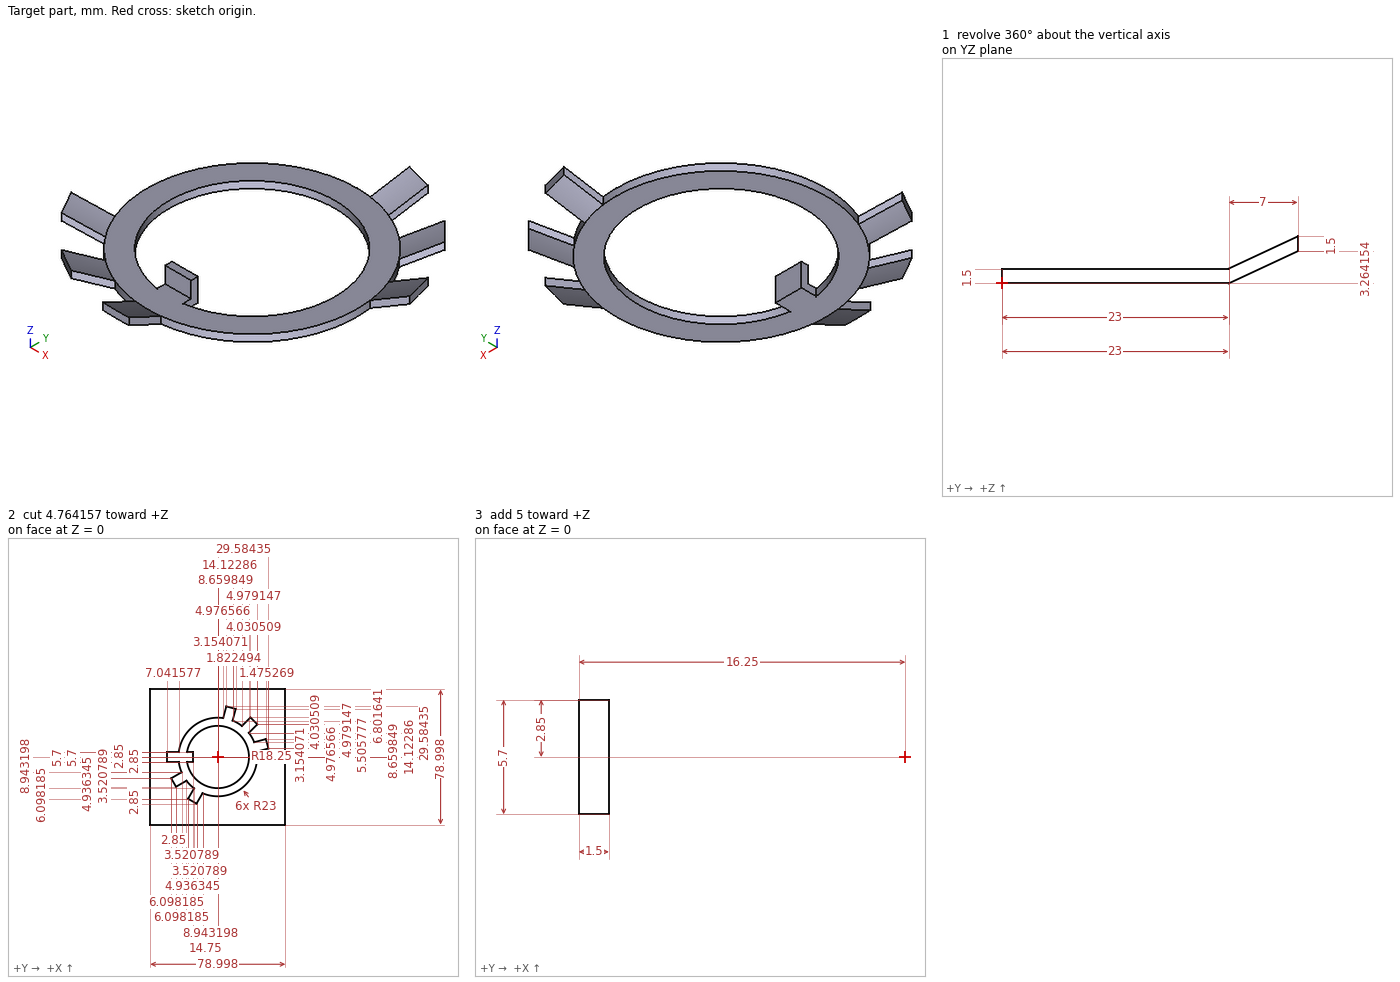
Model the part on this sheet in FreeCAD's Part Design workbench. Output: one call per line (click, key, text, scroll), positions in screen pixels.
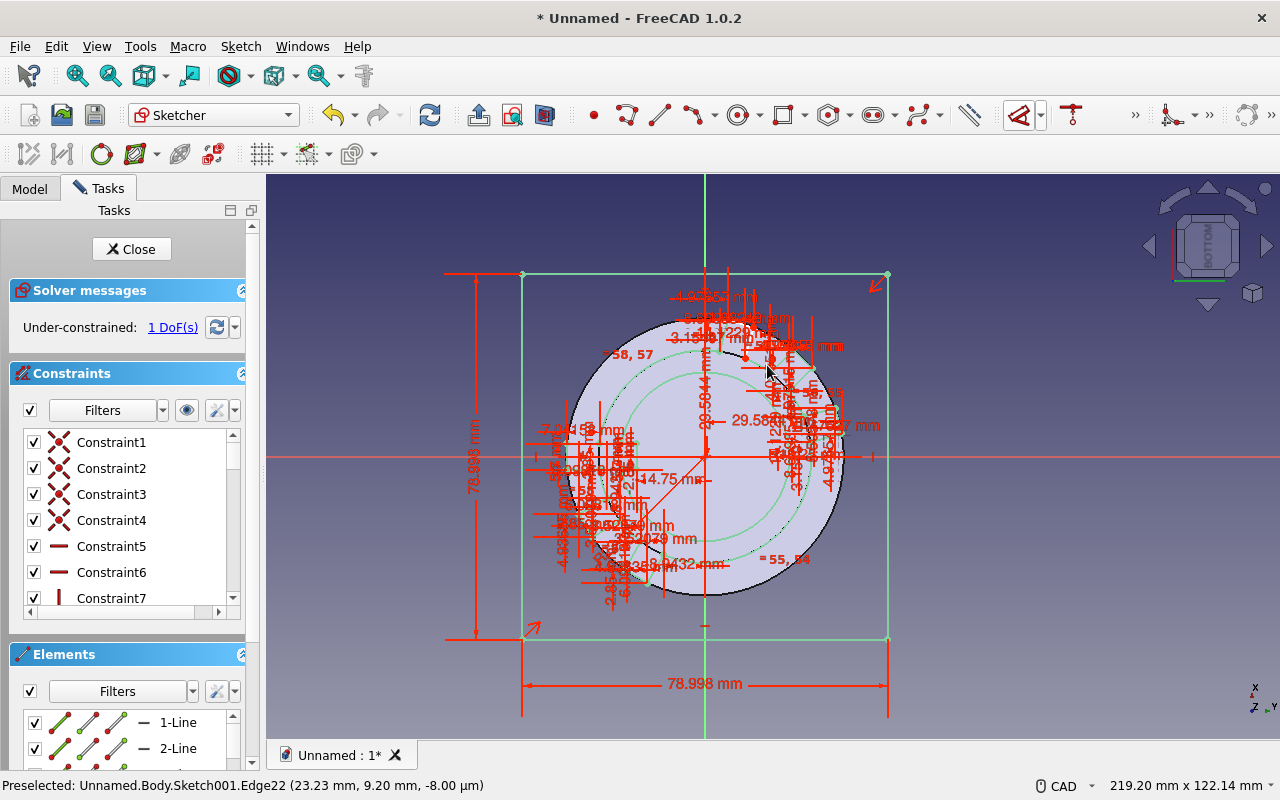
scroll(748, 349, up, 2)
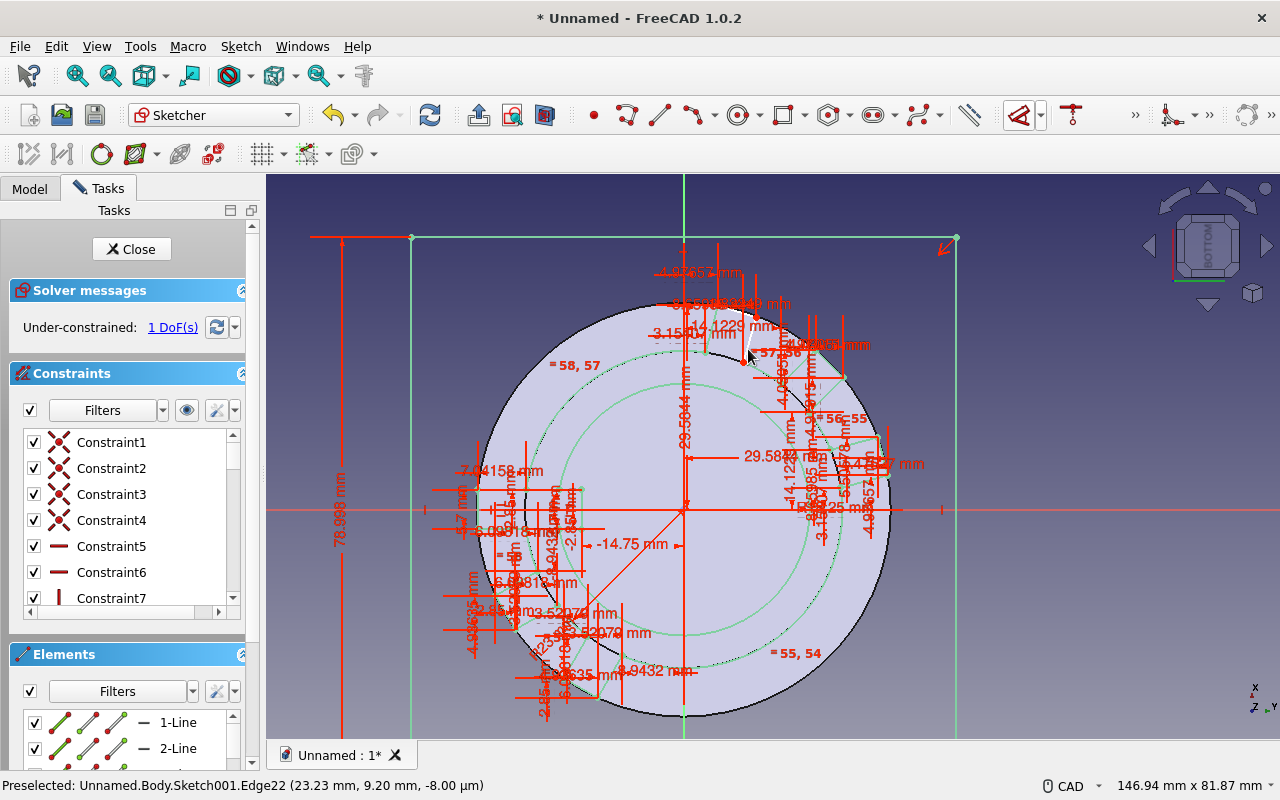
click(747, 349)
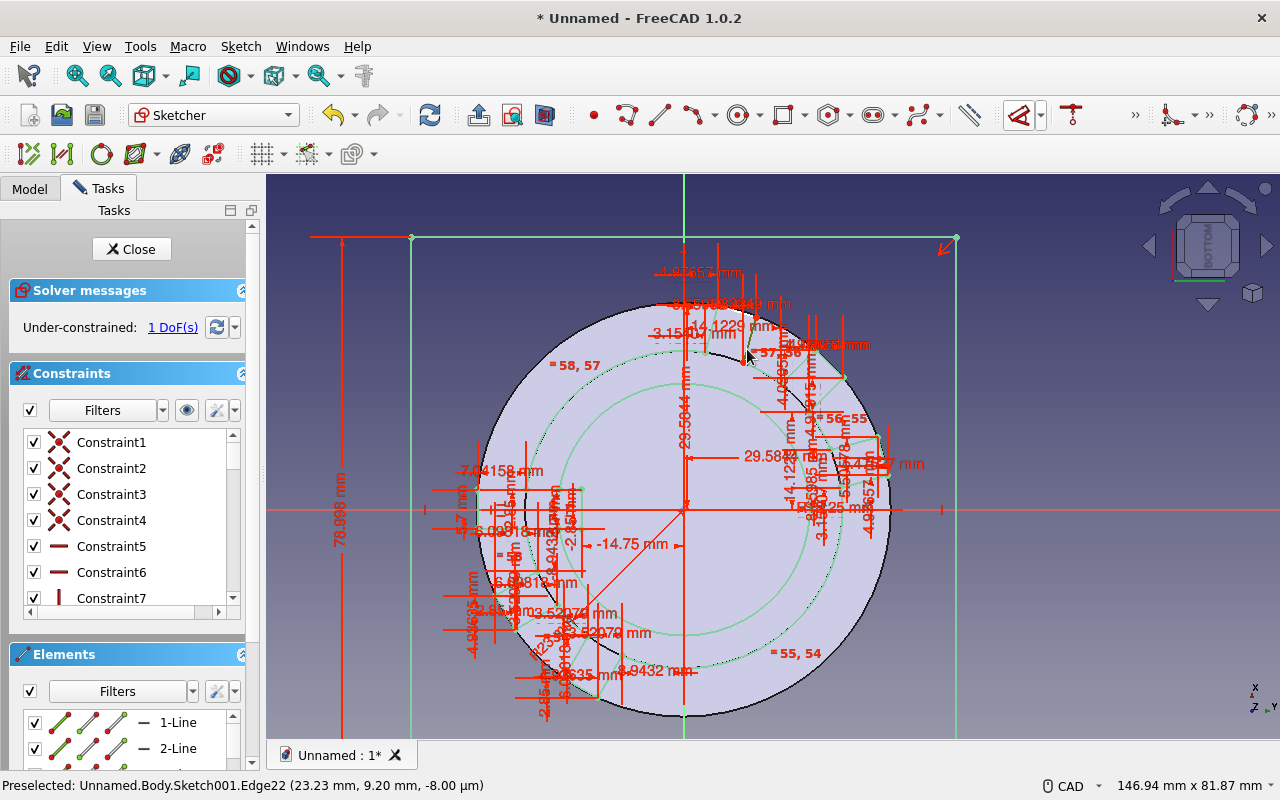
key(i)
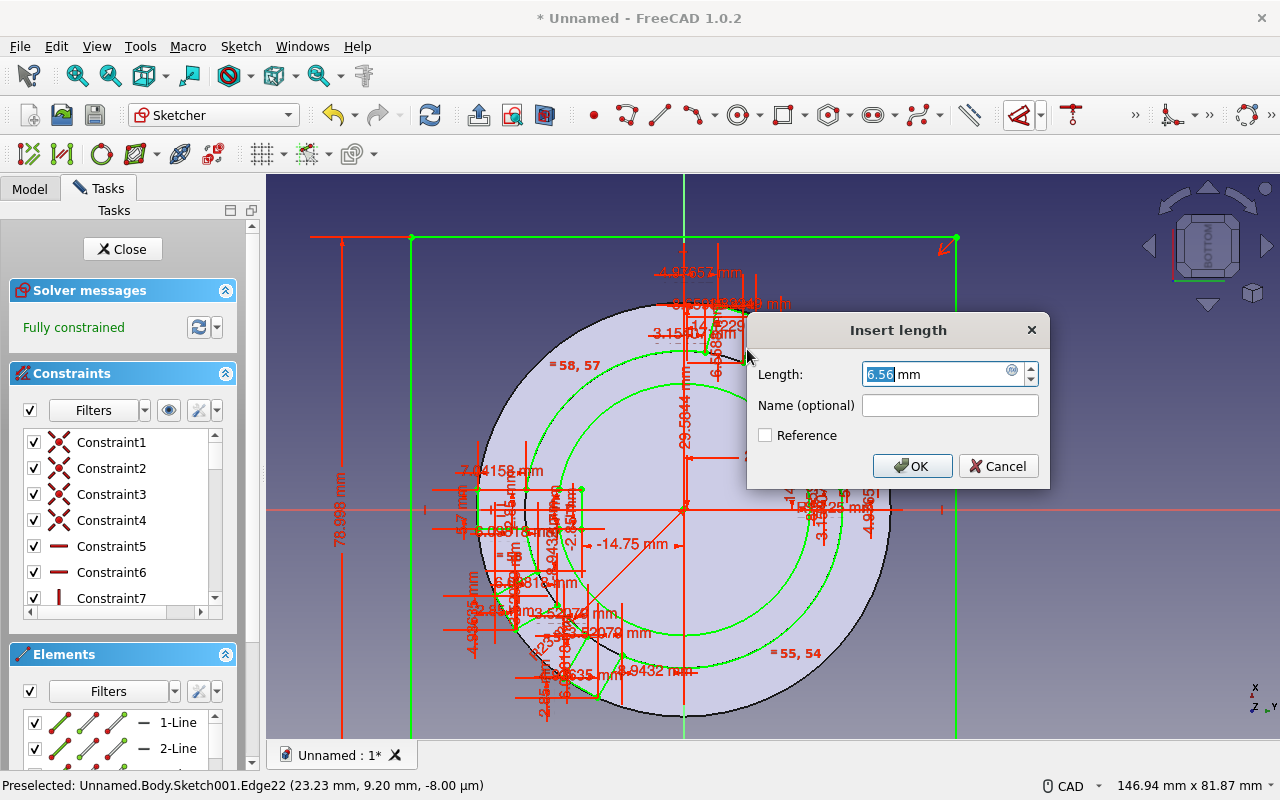
text(6.801641)
key(Return)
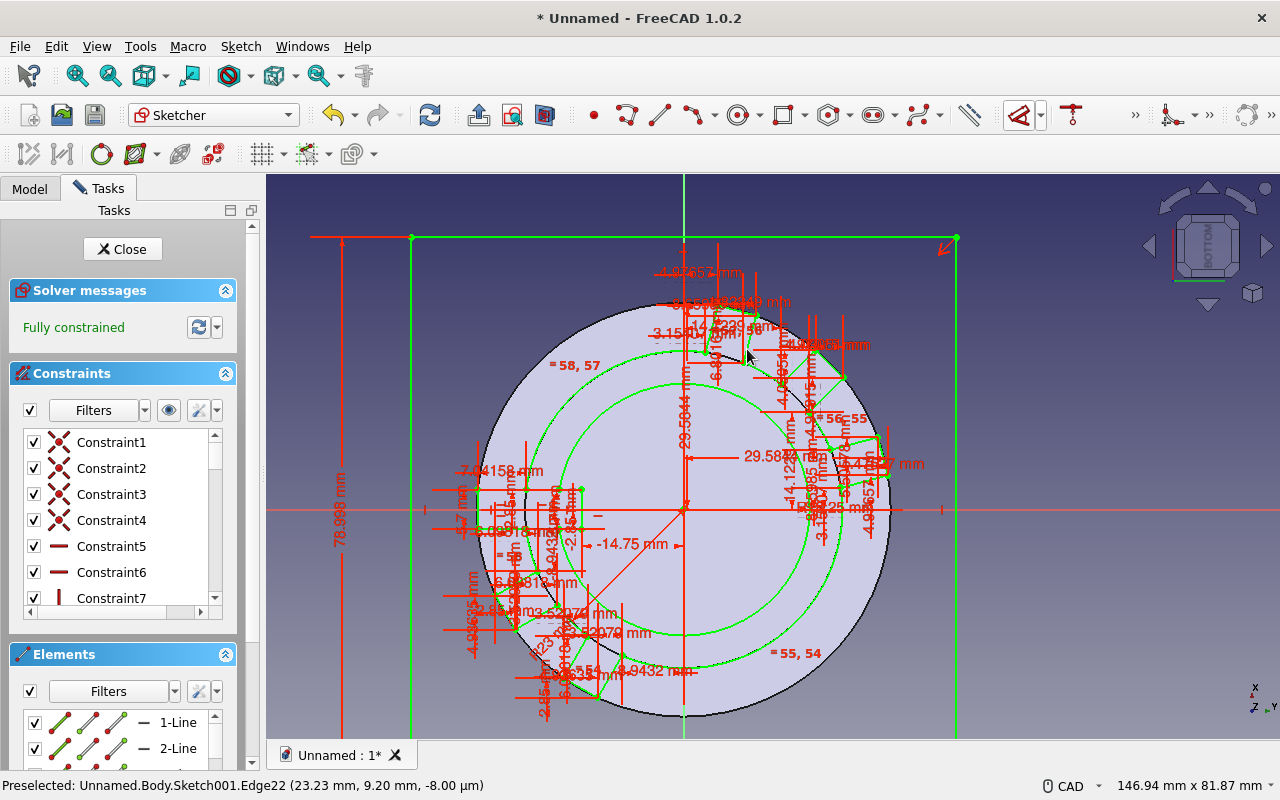
click(123, 249)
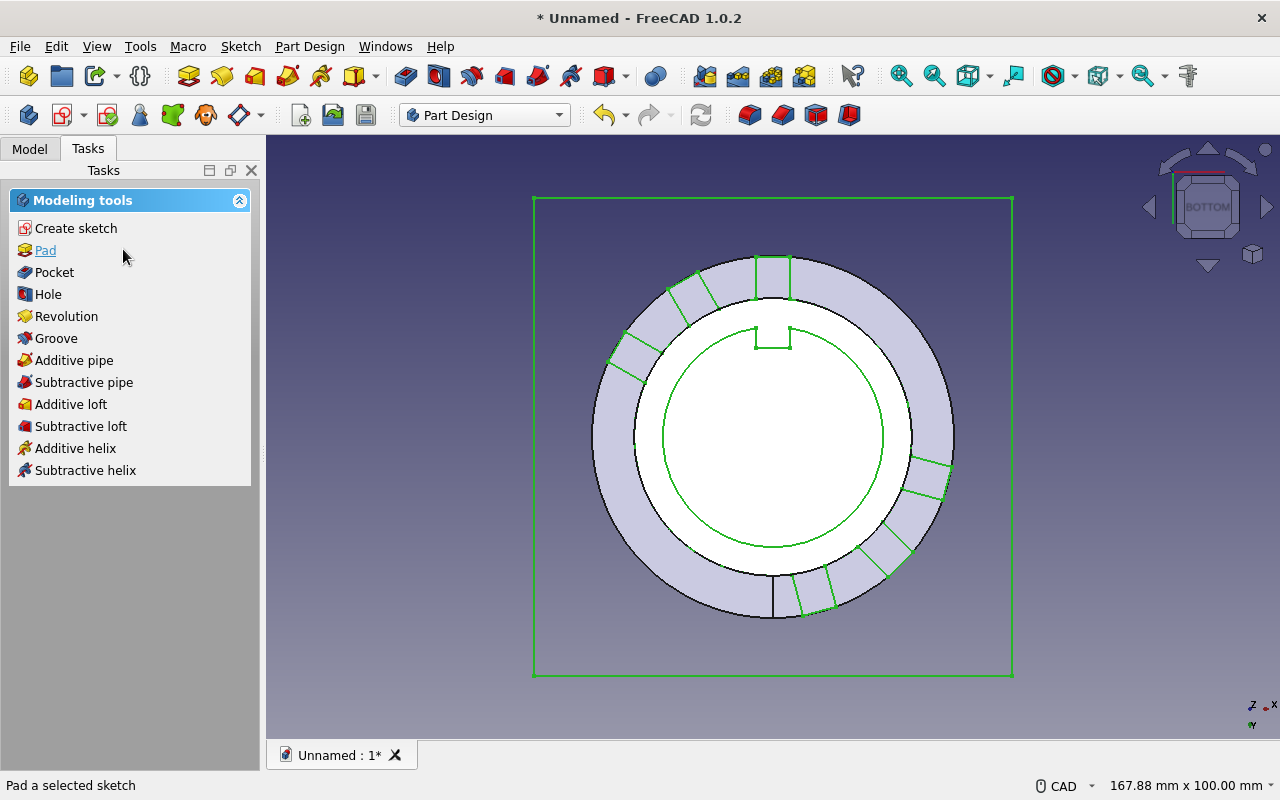
click(406, 76)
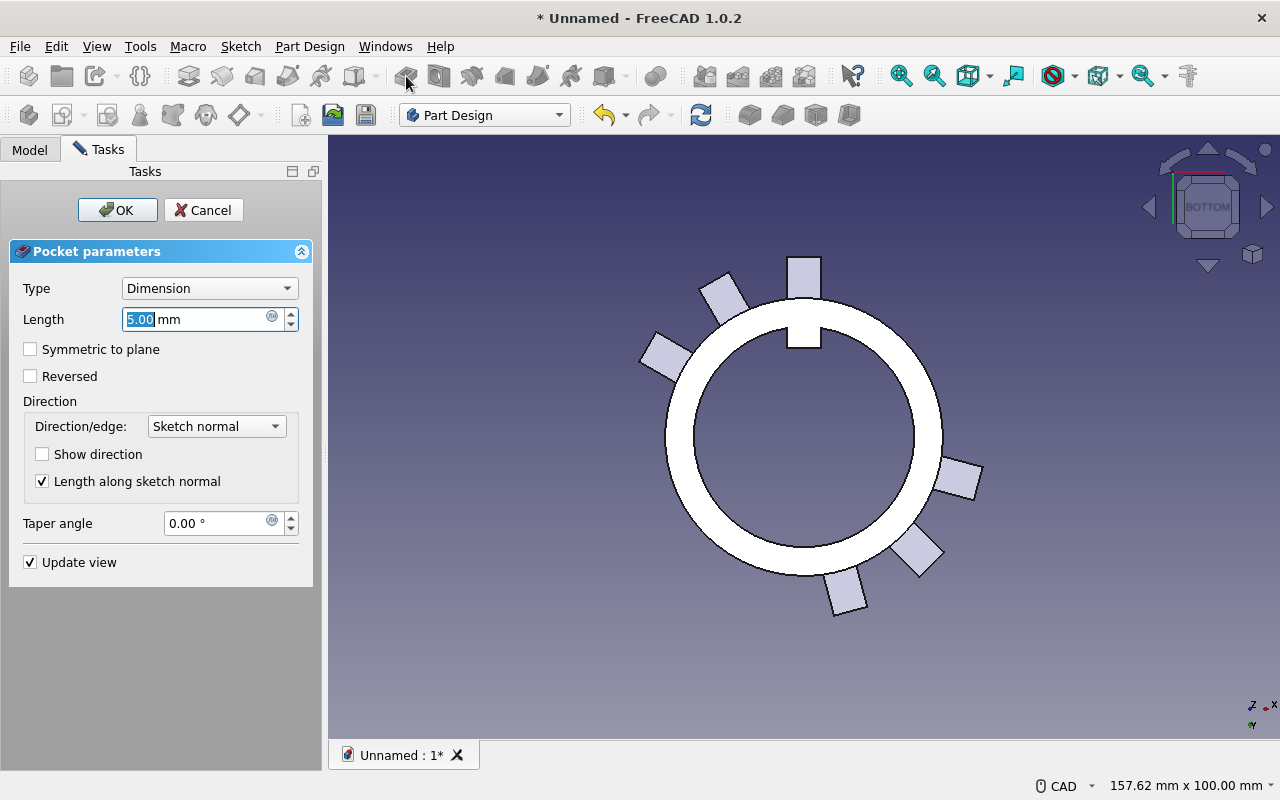
text(4.764157)
key(Tab)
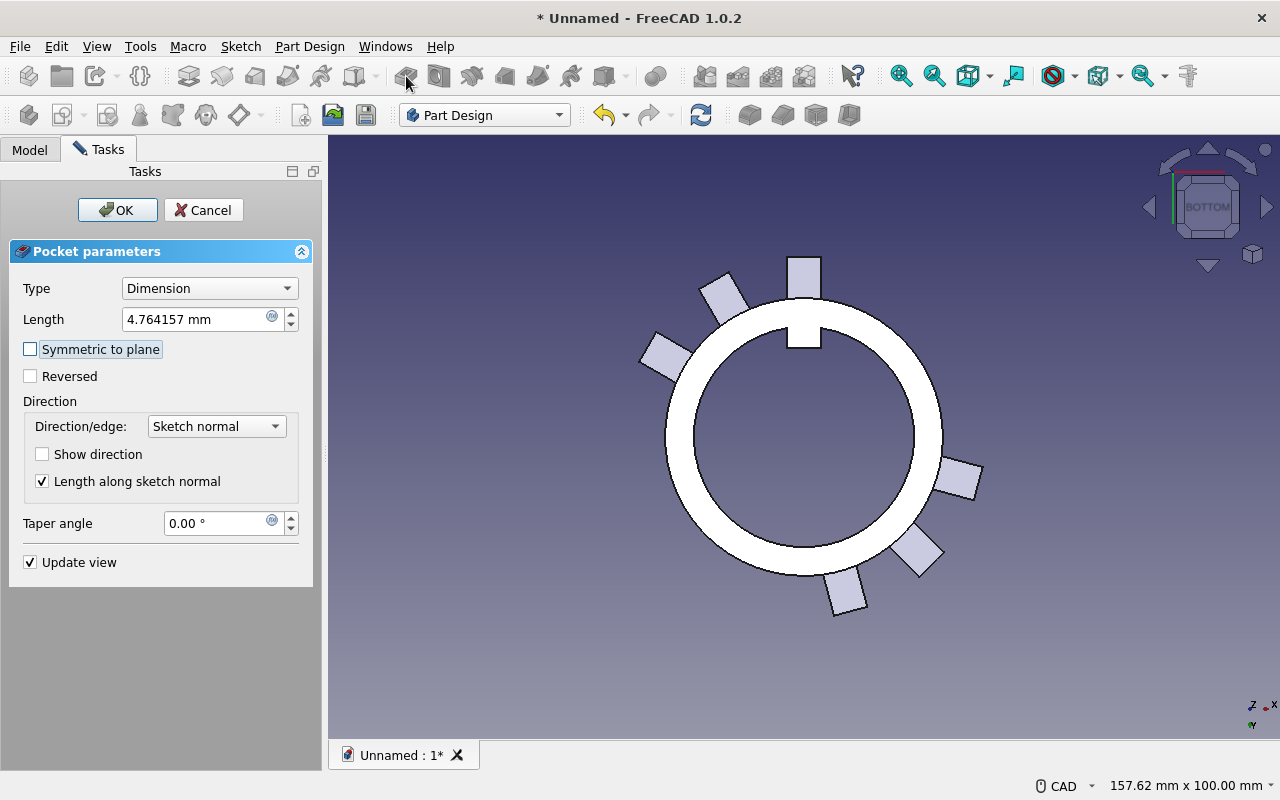
click(118, 210)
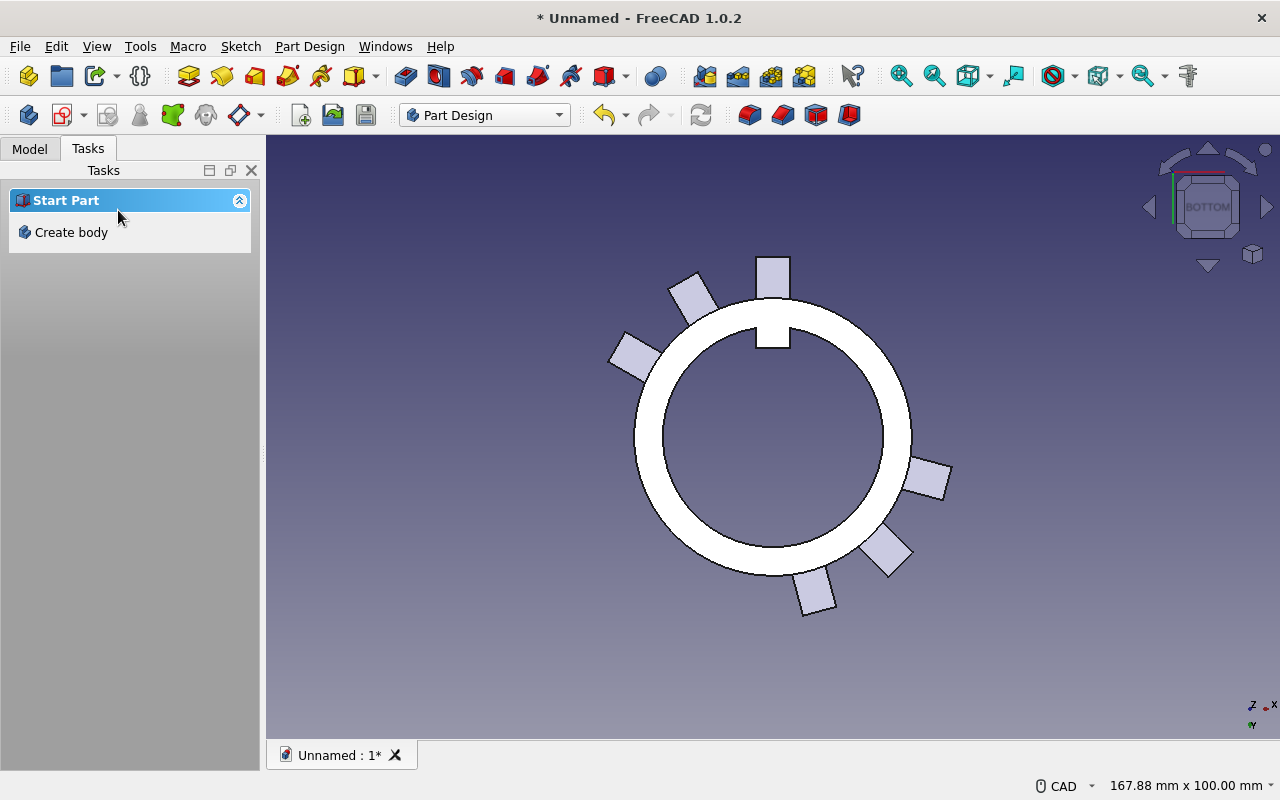
click(773, 317)